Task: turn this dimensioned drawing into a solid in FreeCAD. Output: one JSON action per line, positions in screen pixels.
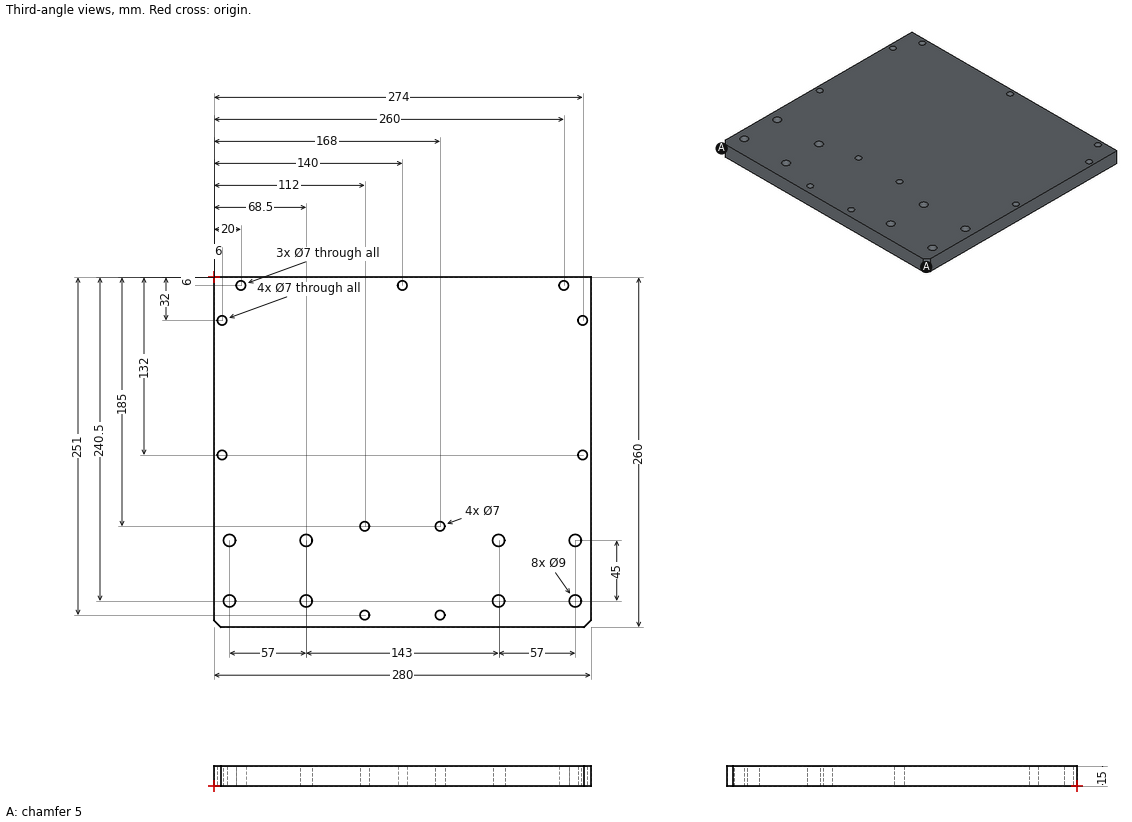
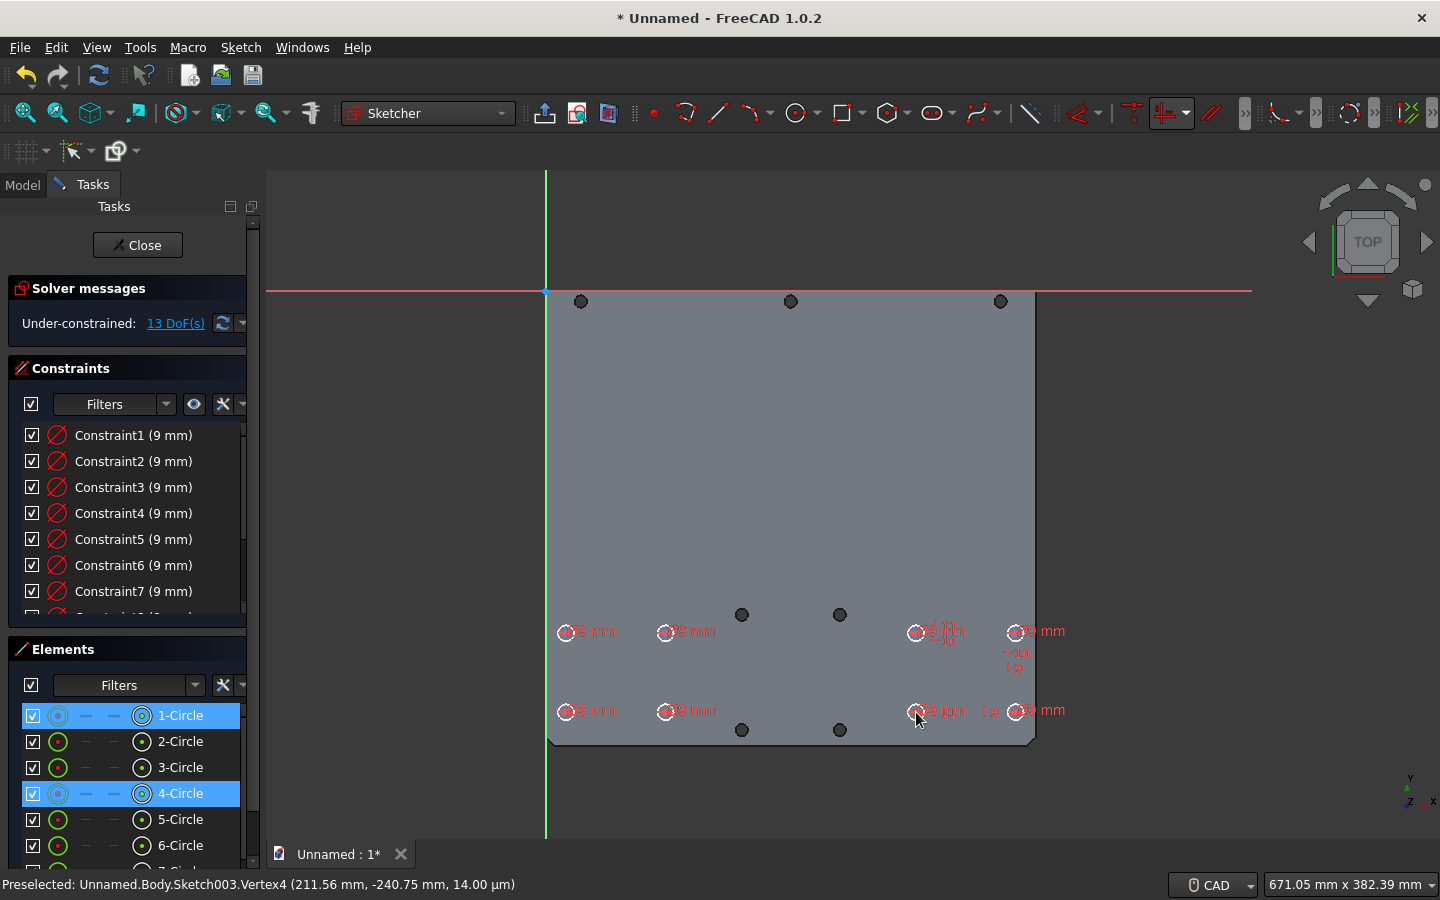
{"action": "left_click", "coordinate": [1188, 114]}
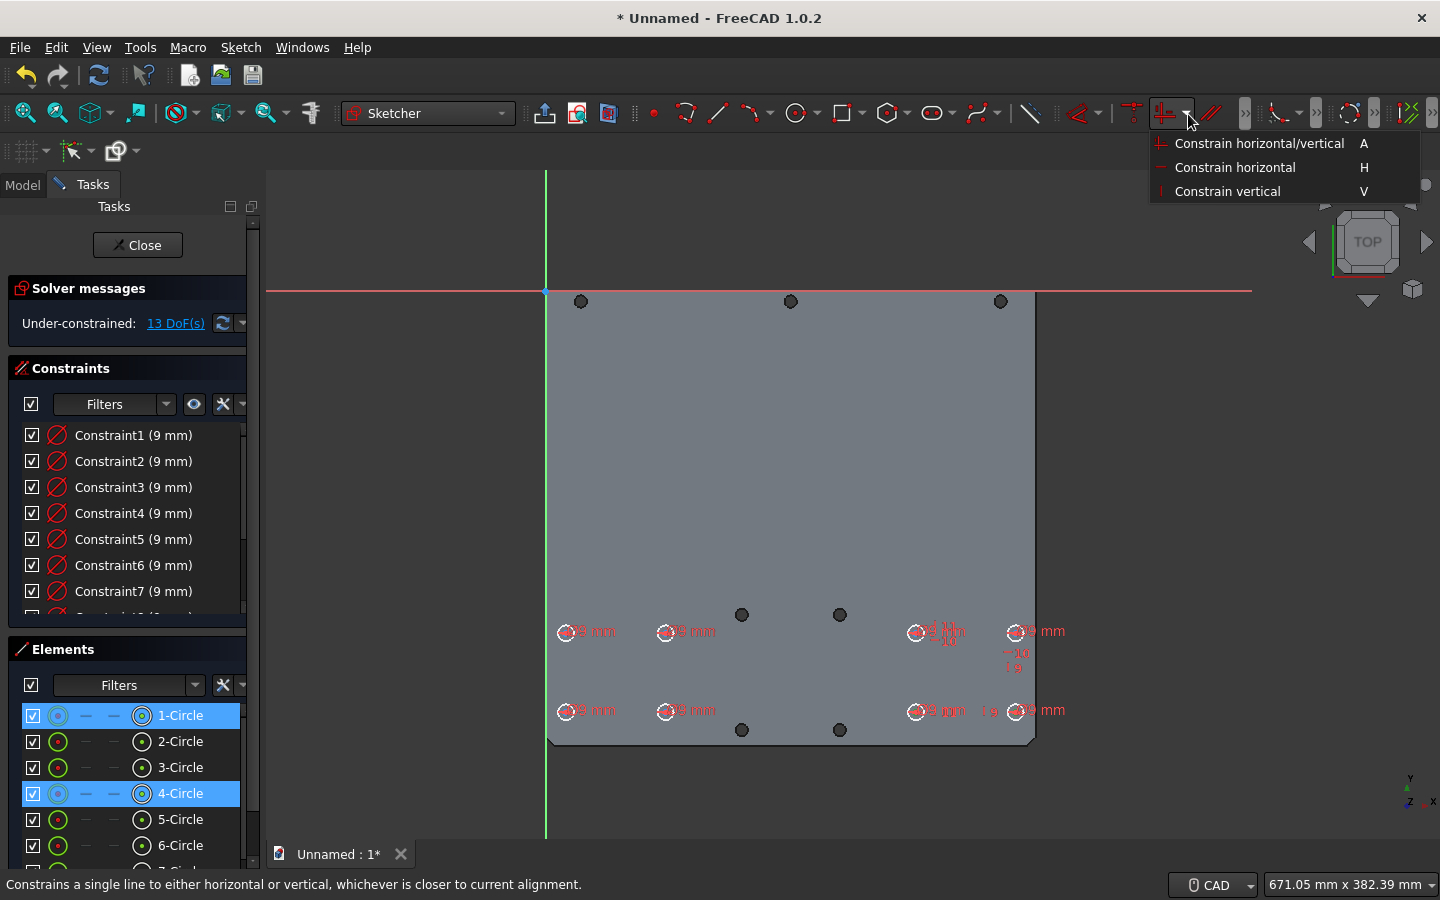
{"action": "left_click", "coordinate": [1285, 167]}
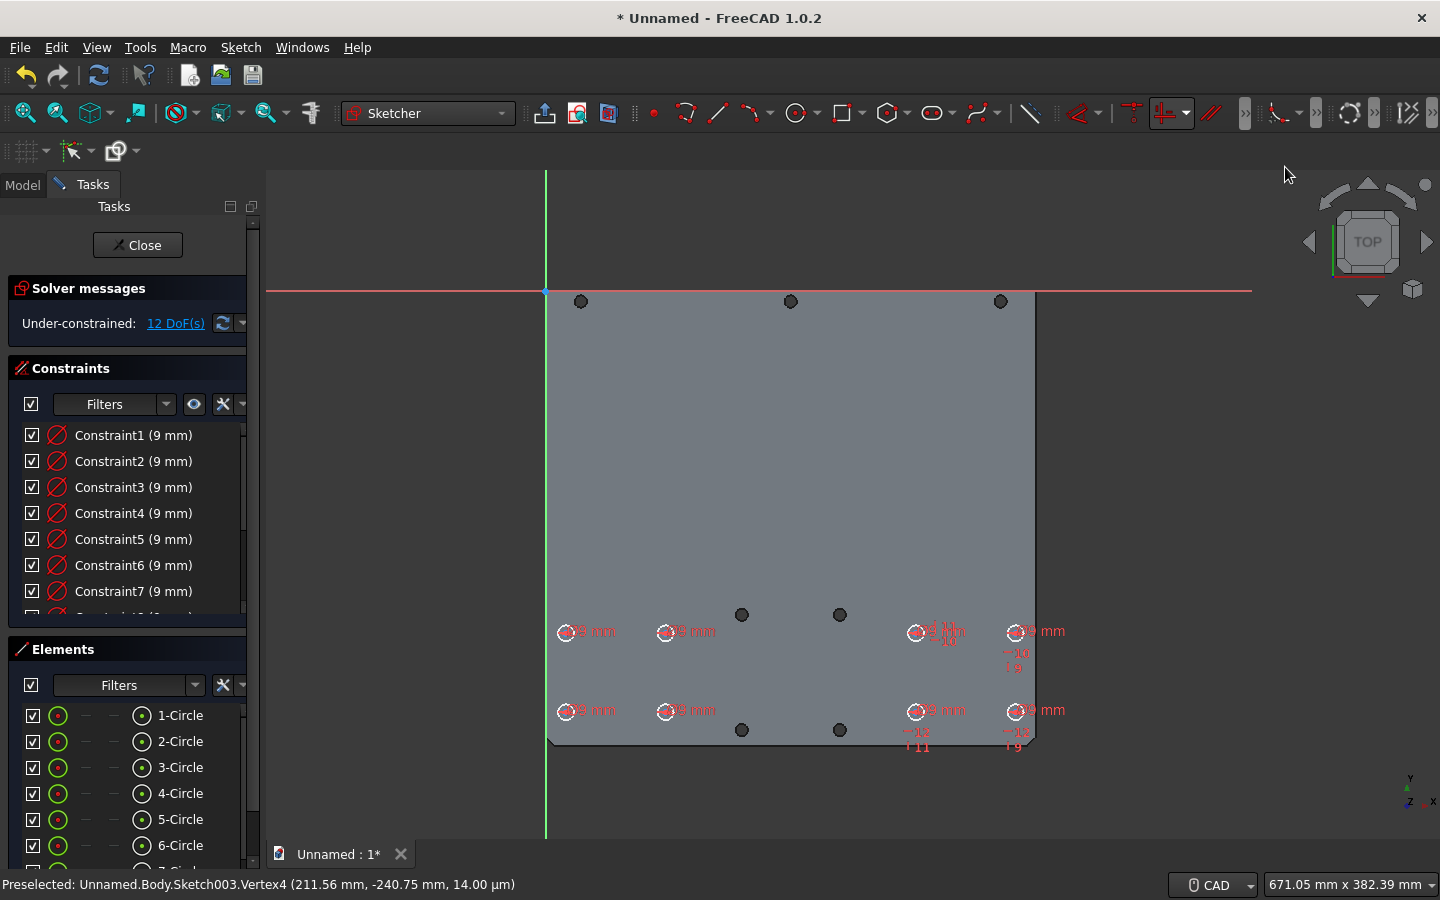
{"action": "left_click", "coordinate": [916, 712]}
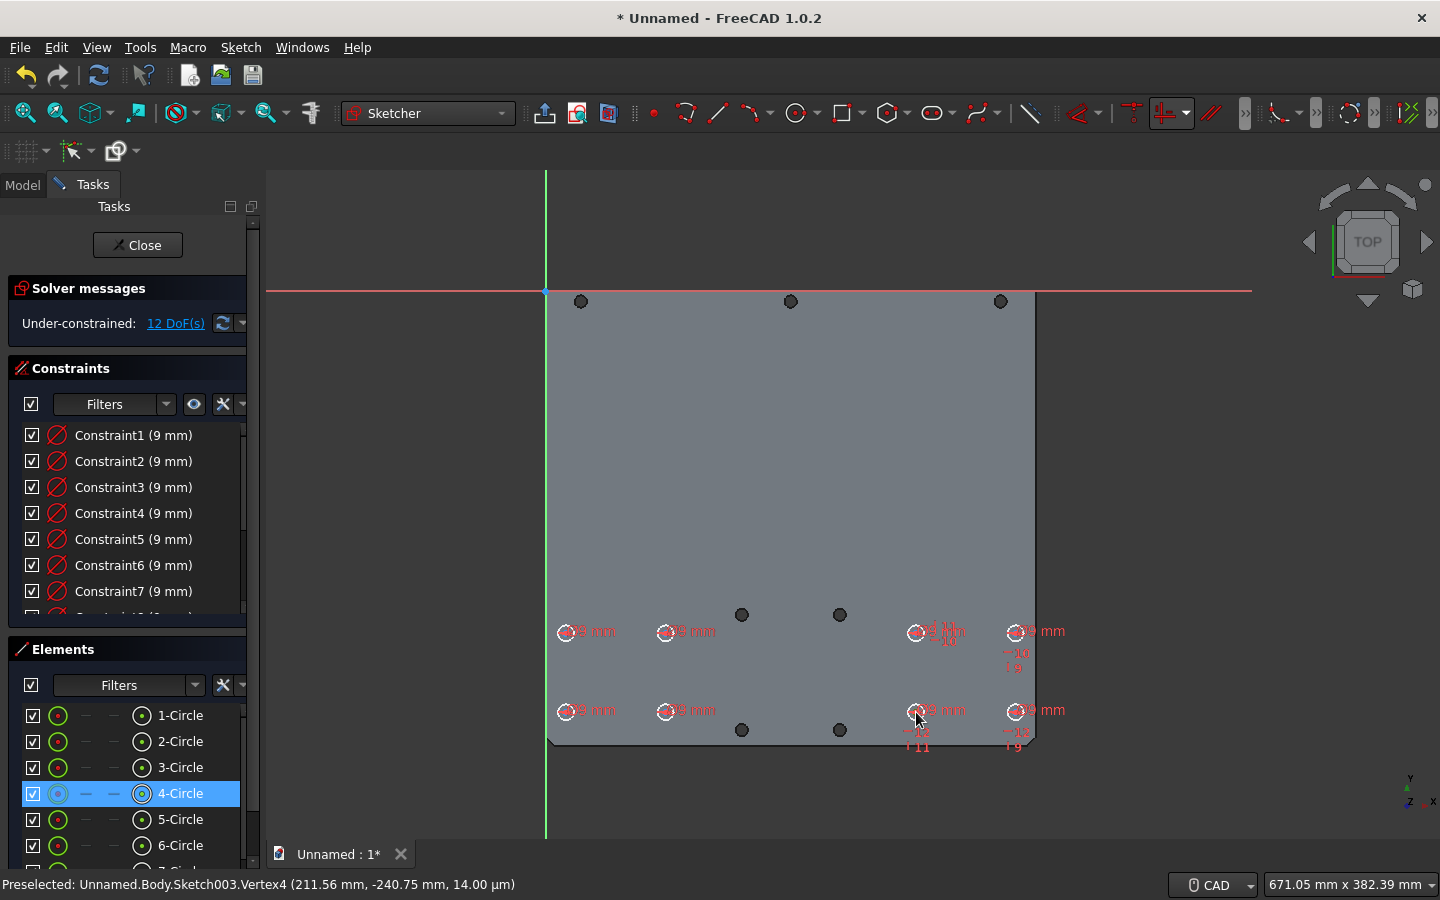
{"action": "left_click", "coordinate": [666, 712]}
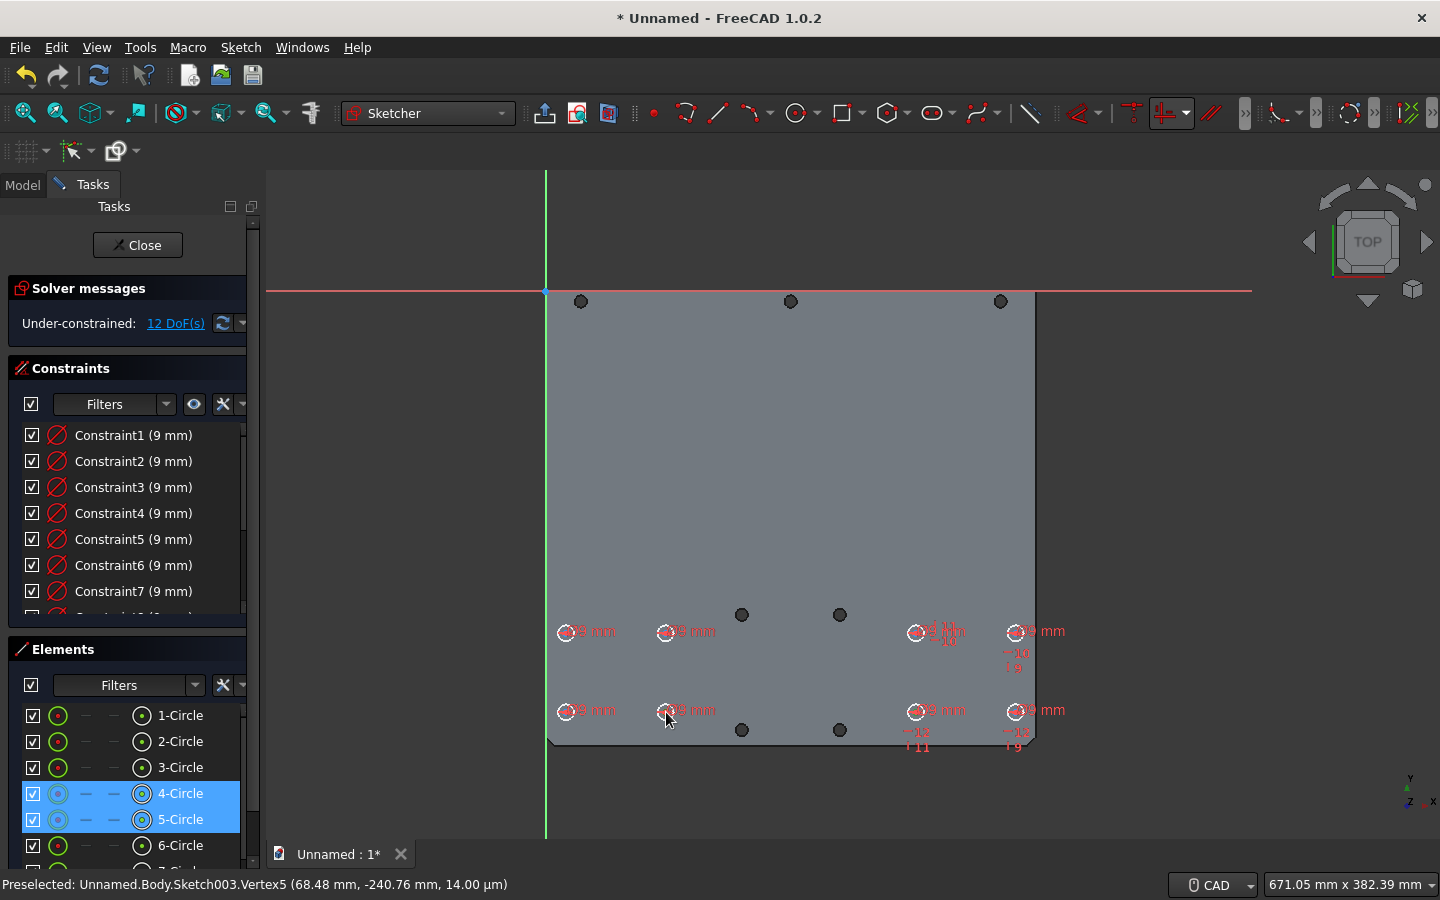
{"action": "left_click", "coordinate": [1188, 114]}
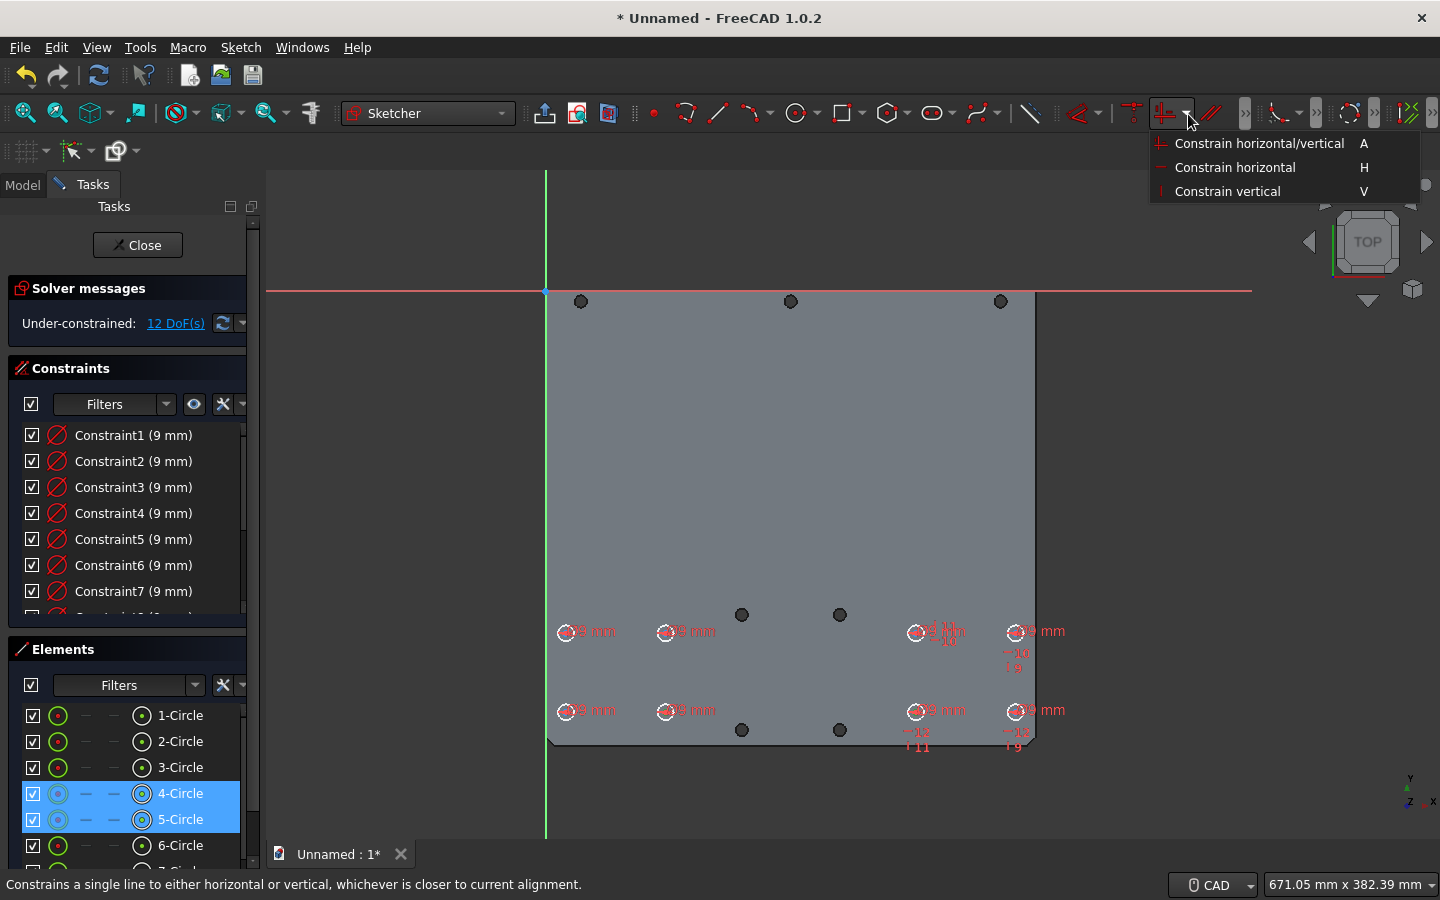
{"action": "left_click", "coordinate": [1285, 167]}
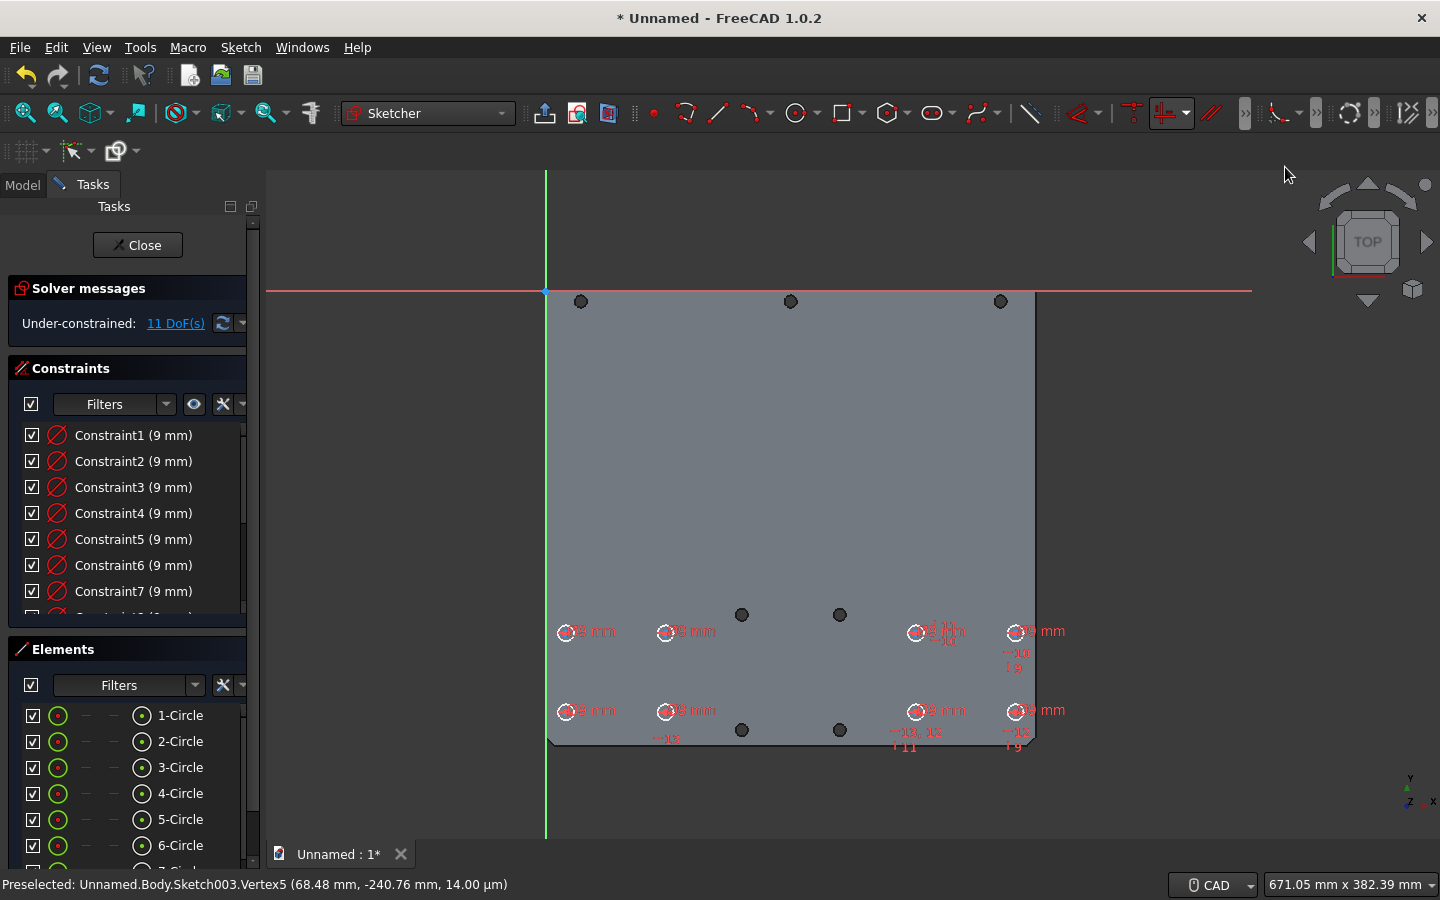
{"action": "left_click", "coordinate": [666, 712]}